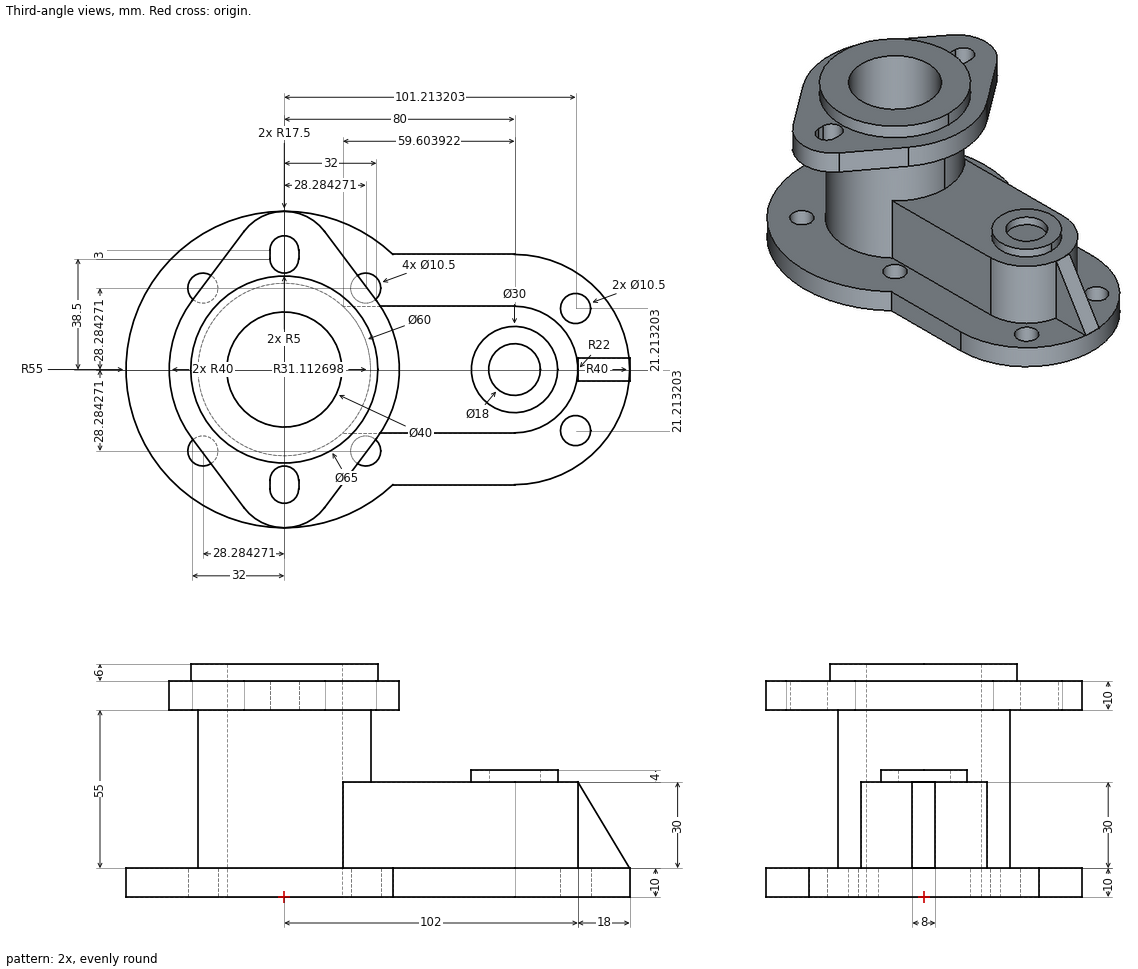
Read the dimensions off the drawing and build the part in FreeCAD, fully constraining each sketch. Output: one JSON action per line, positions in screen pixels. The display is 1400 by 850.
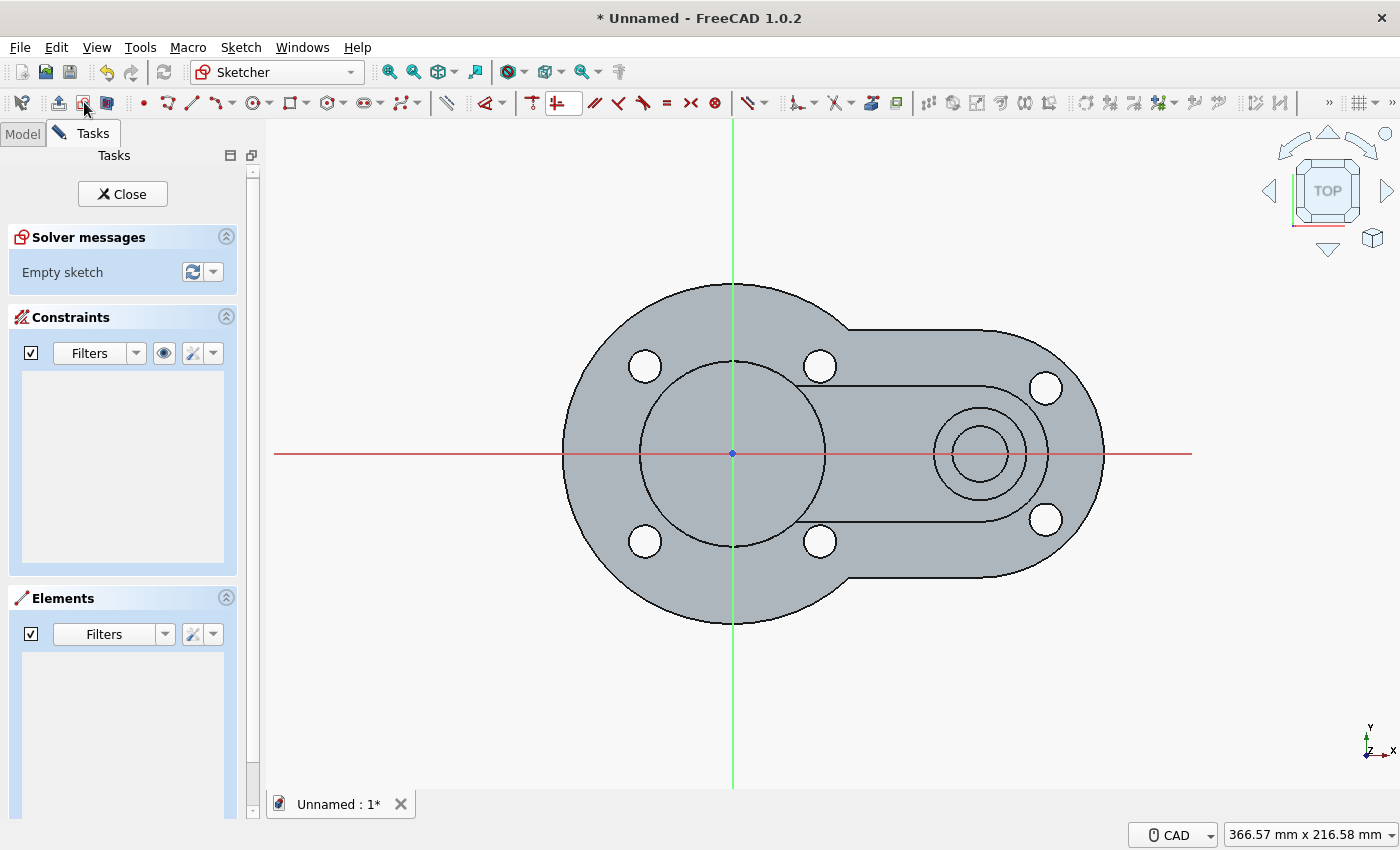
{"action": "key", "text": "g l"}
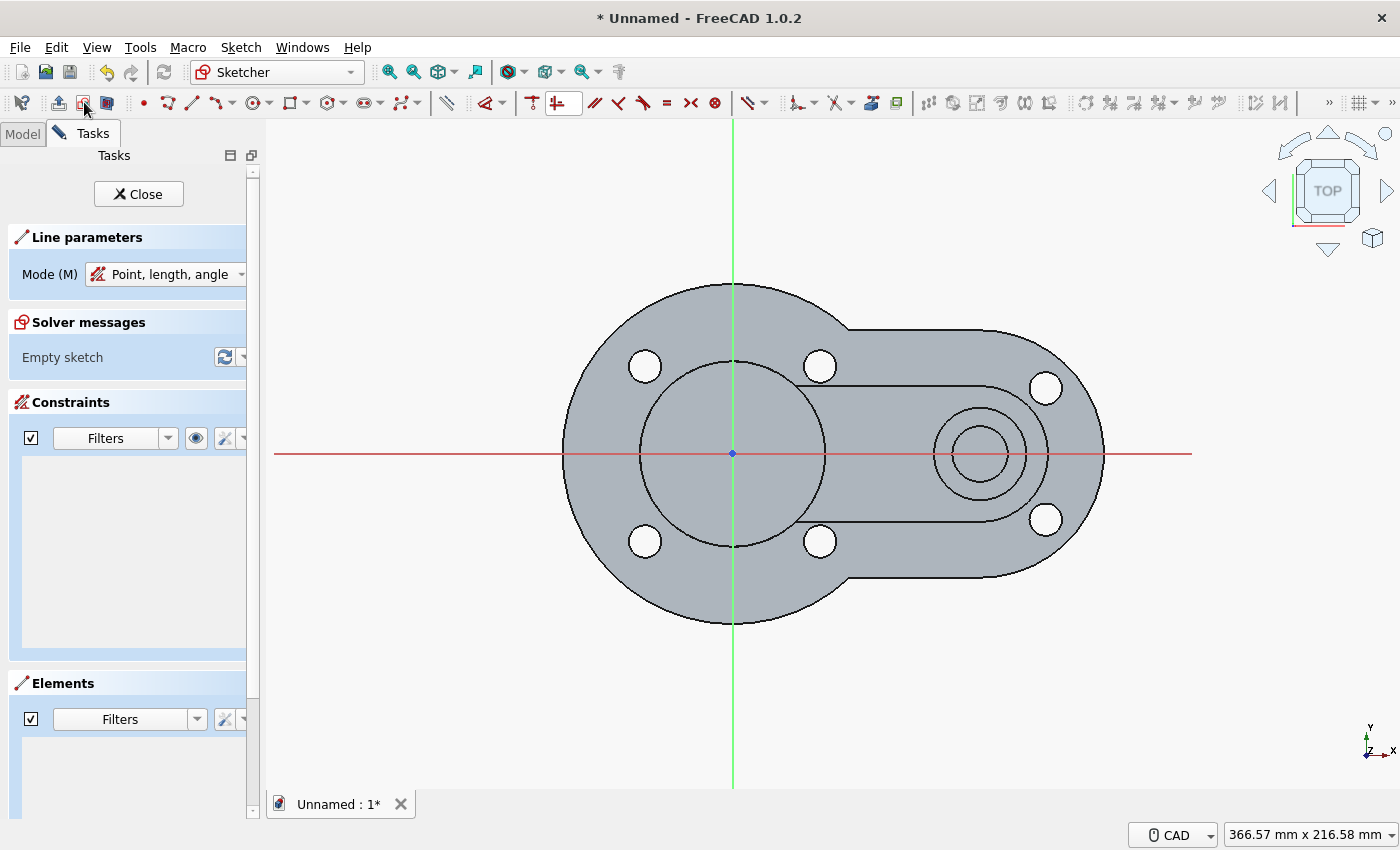
{"action": "left_click", "coordinate": [832, 380]}
{"action": "left_click", "coordinate": [776, 306]}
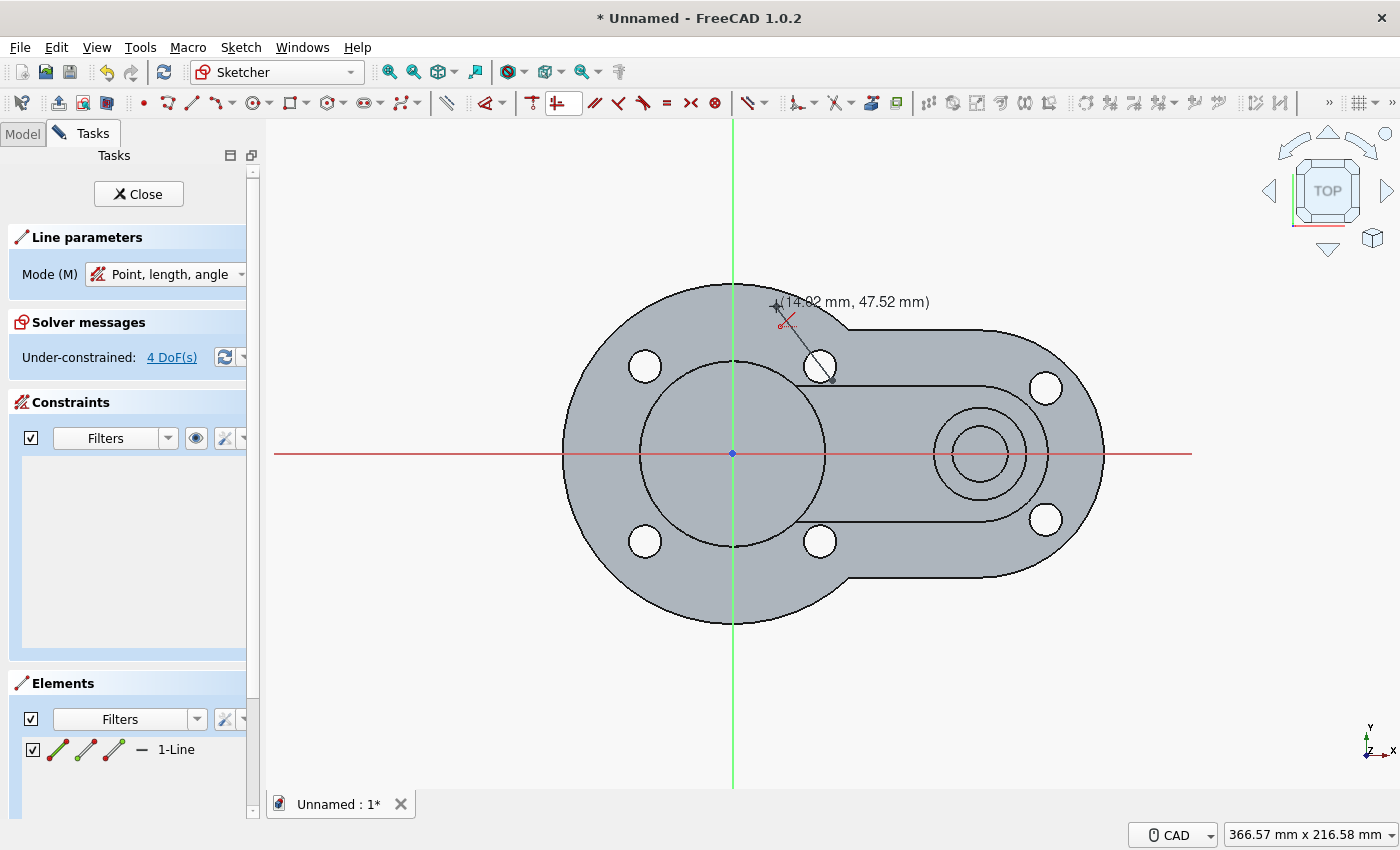
{"action": "left_click", "coordinate": [689, 306]}
{"action": "left_click", "coordinate": [634, 380]}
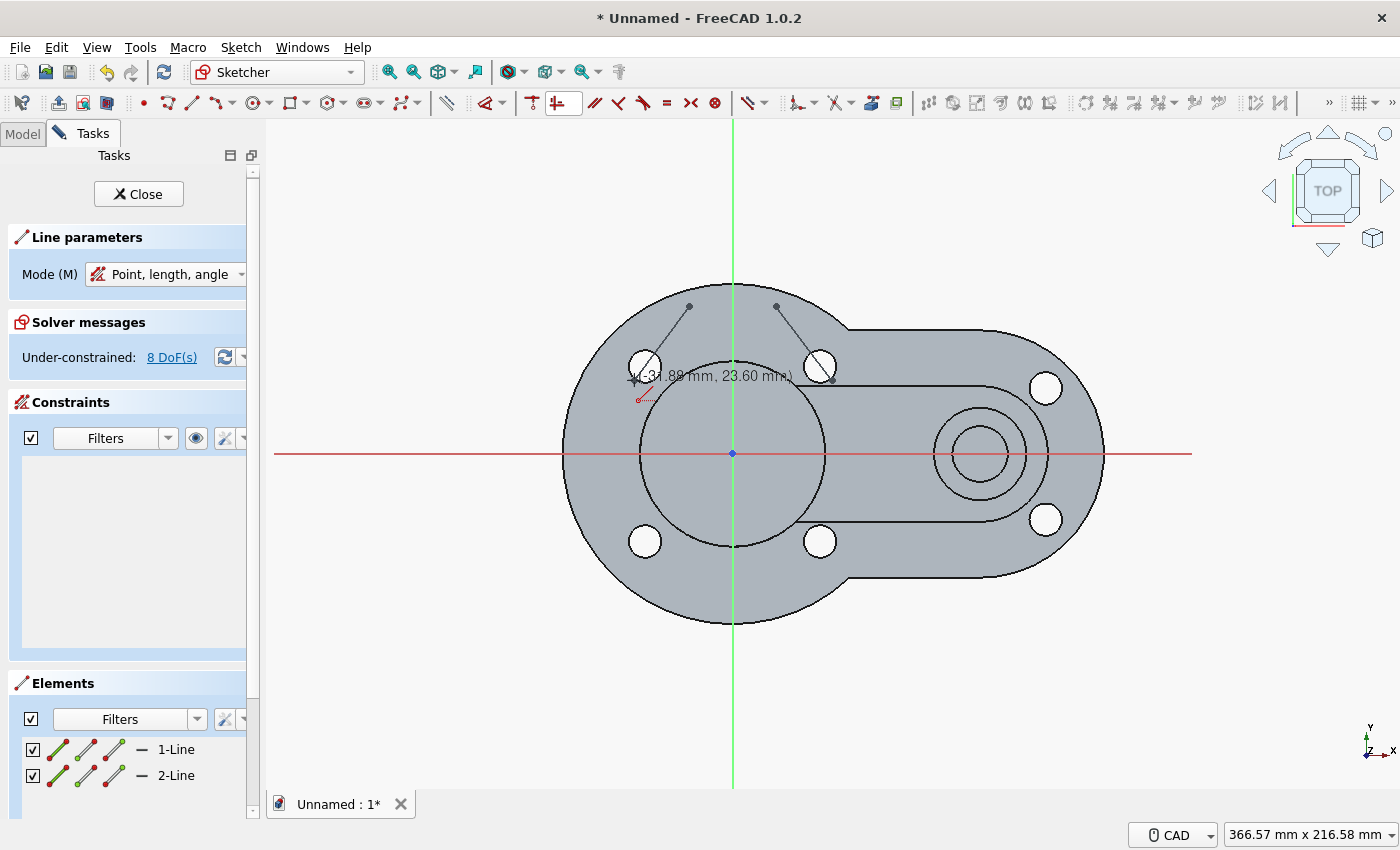
{"action": "left_click", "coordinate": [634, 528]}
{"action": "left_click", "coordinate": [689, 602]}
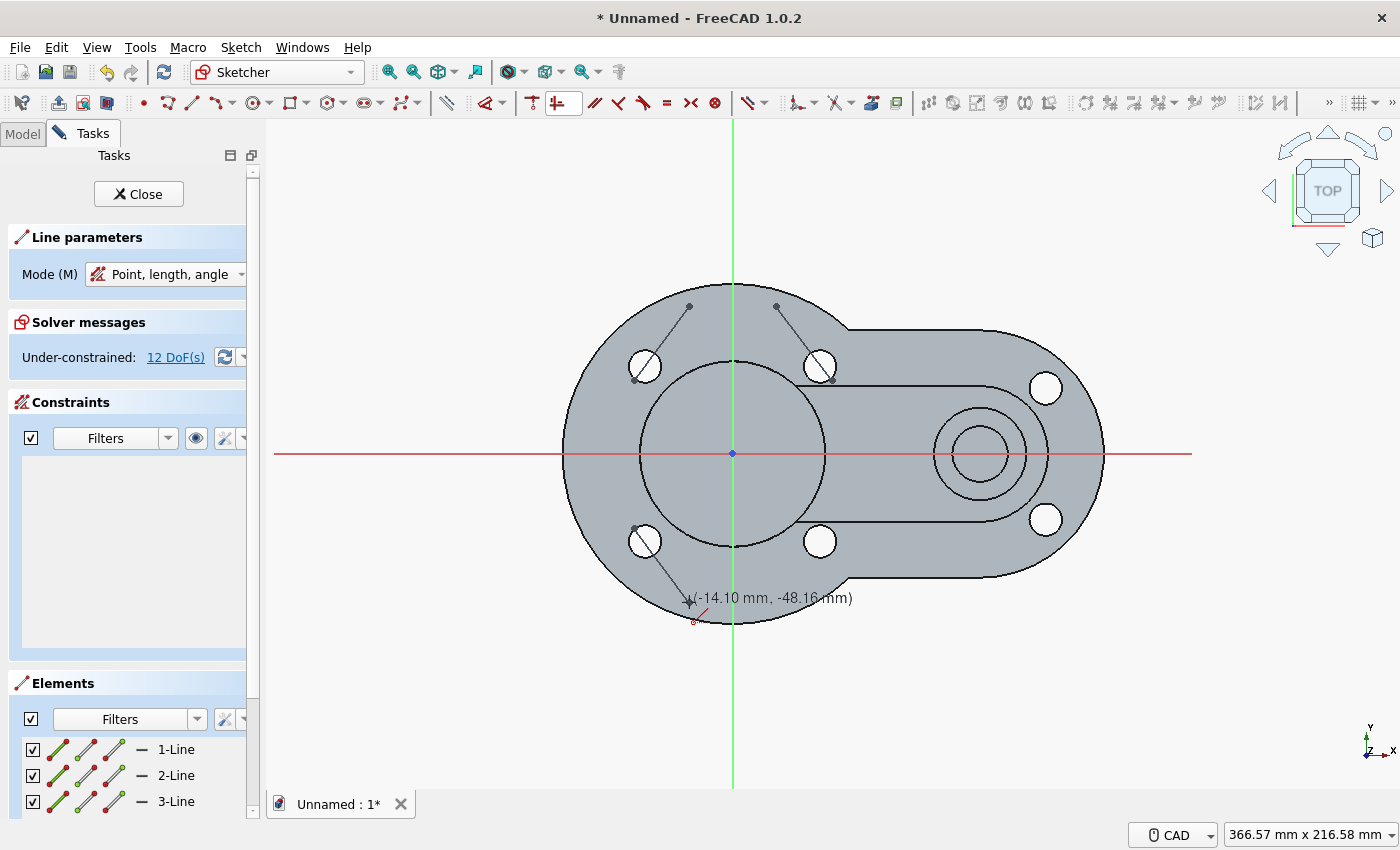
{"action": "left_click", "coordinate": [776, 602]}
{"action": "left_click", "coordinate": [832, 528]}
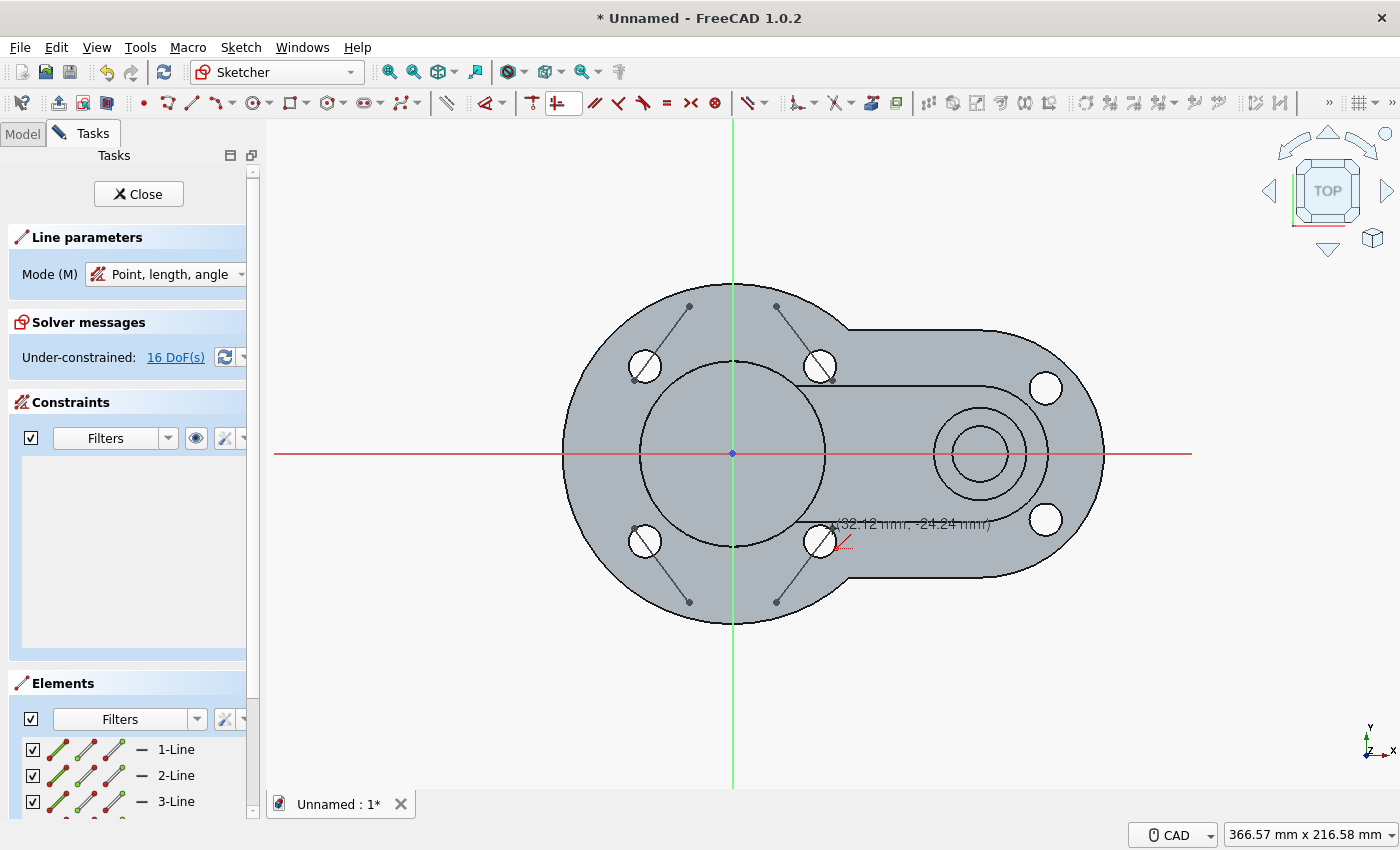
{"action": "key", "text": "g 3 a"}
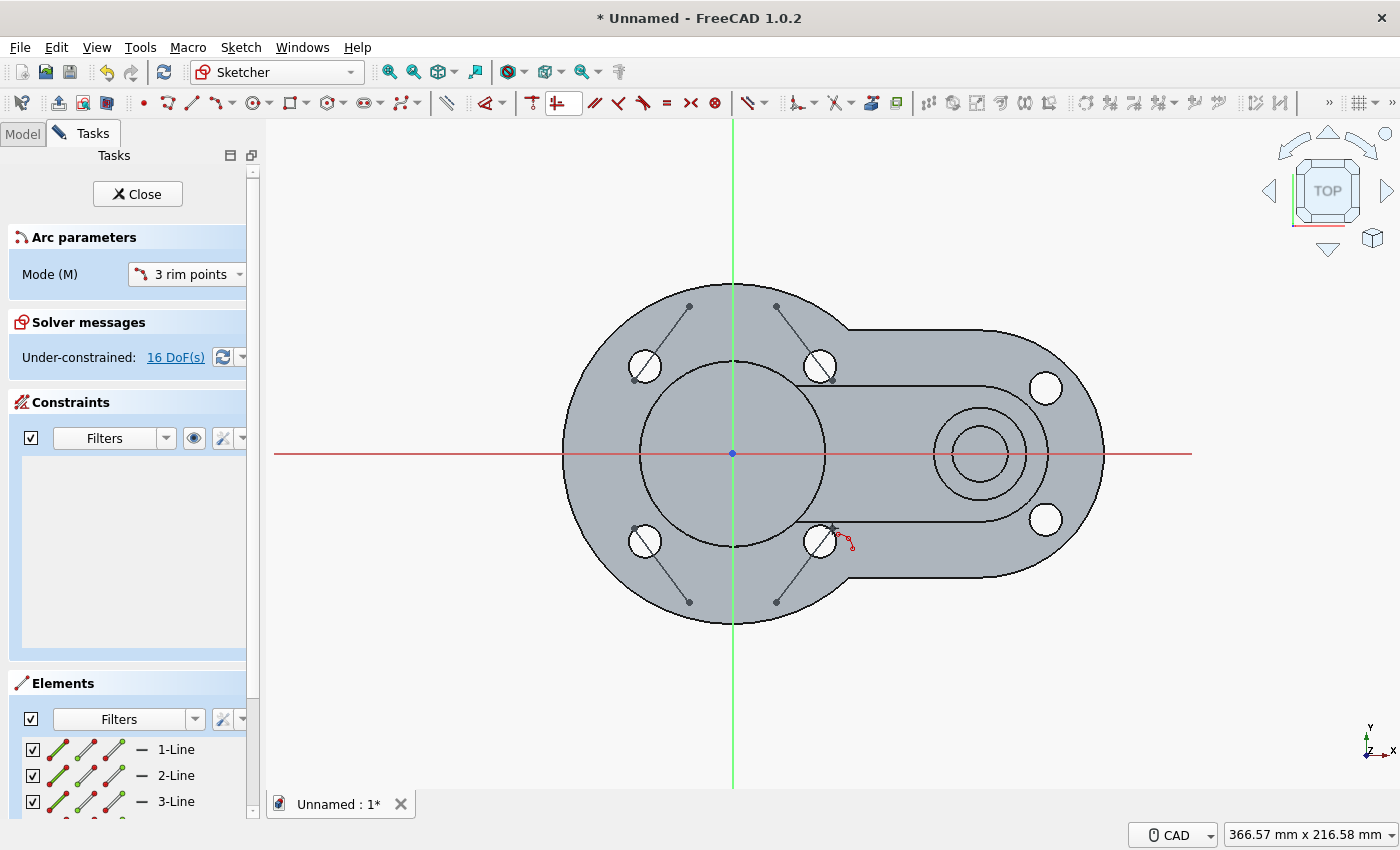
{"action": "left_click", "coordinate": [776, 307]}
{"action": "left_click", "coordinate": [689, 307]}
{"action": "left_click", "coordinate": [752, 288]}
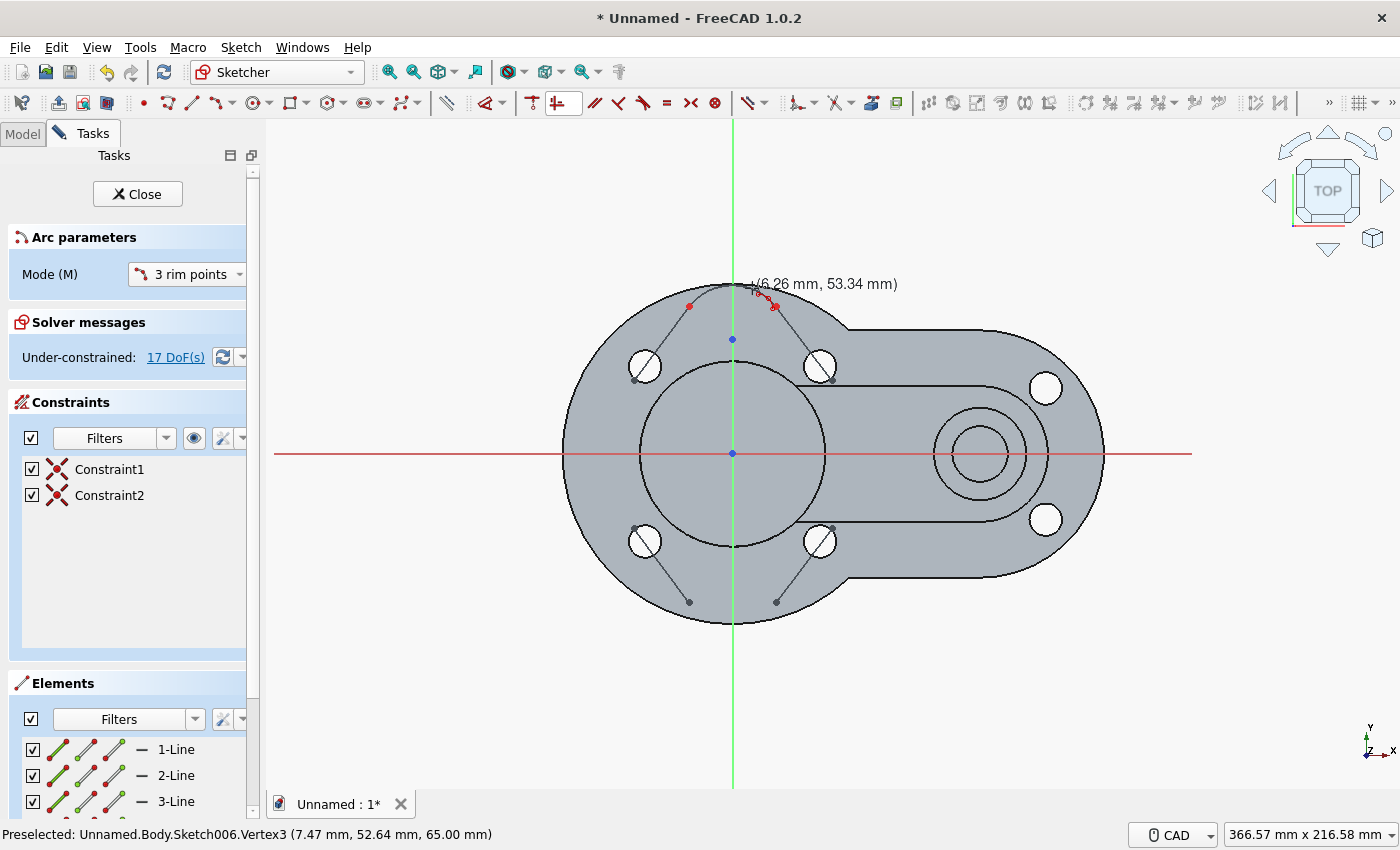
{"action": "left_click", "coordinate": [634, 381]}
{"action": "left_click", "coordinate": [634, 529]}
{"action": "left_click", "coordinate": [610, 438]}